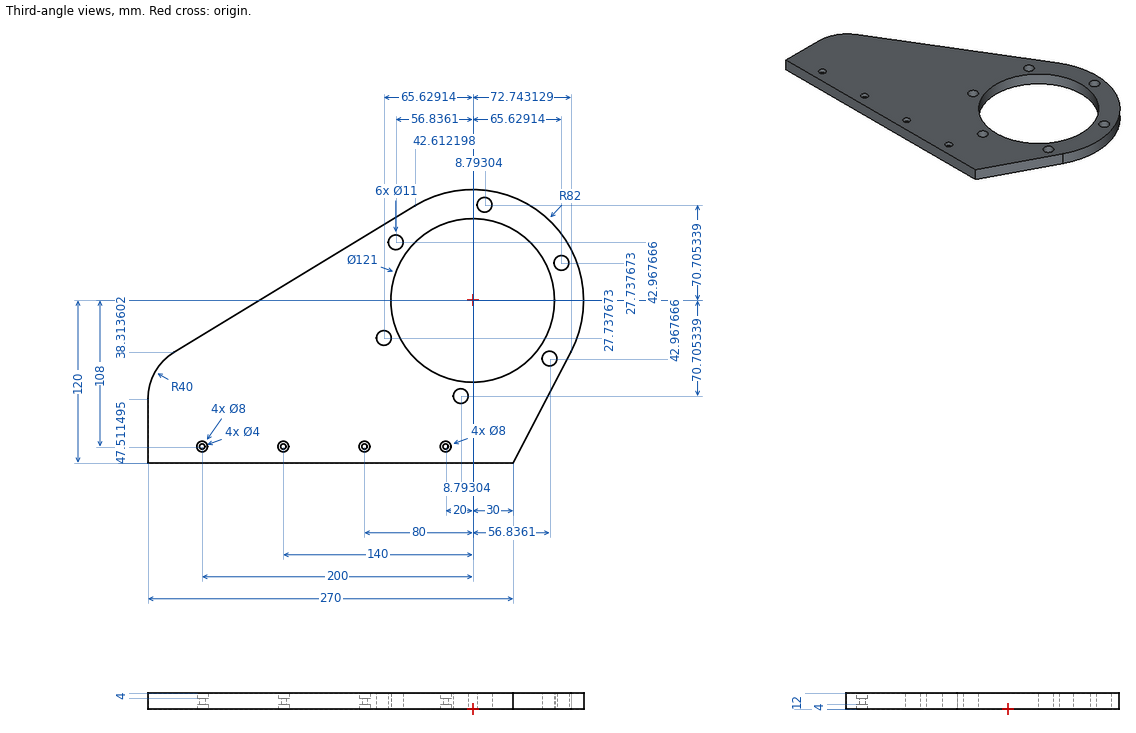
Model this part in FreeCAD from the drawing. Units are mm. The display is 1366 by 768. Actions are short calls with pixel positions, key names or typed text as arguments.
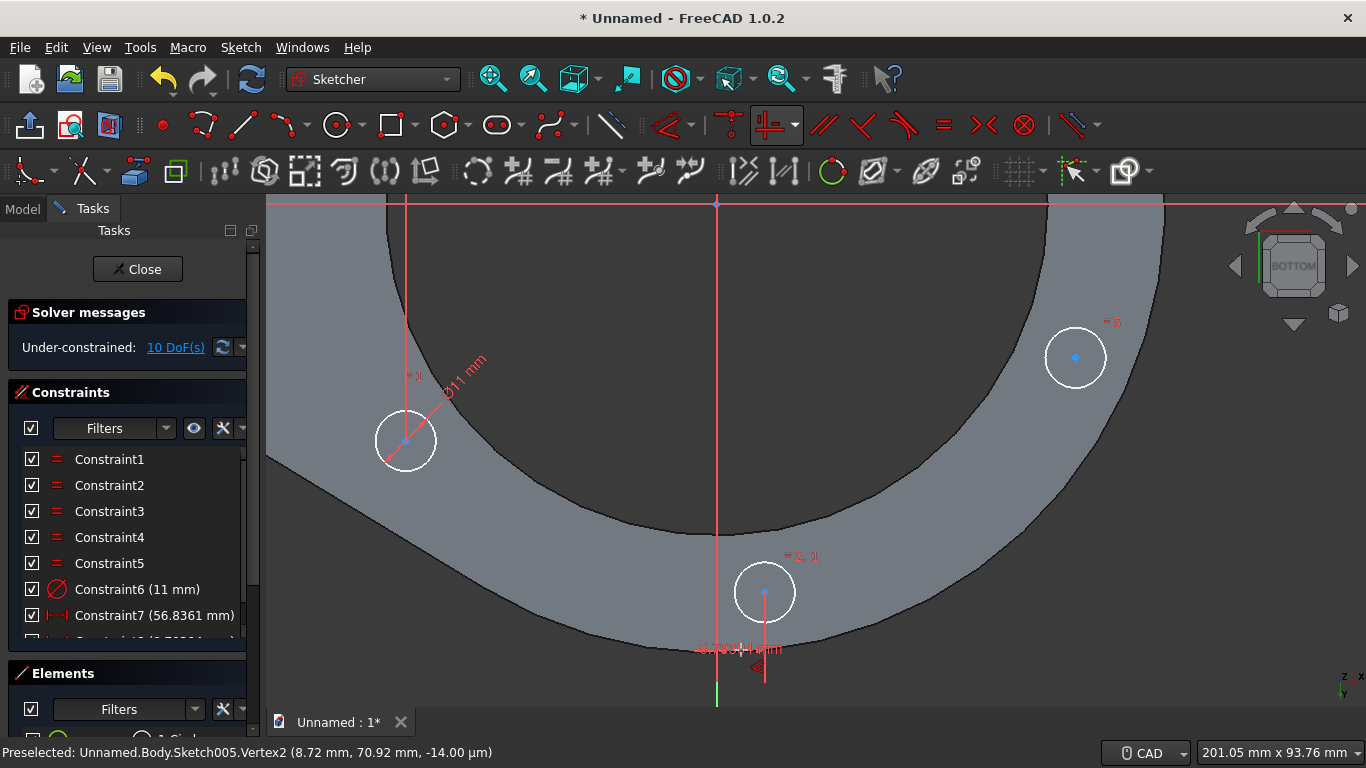
scroll(765, 594, down, 5)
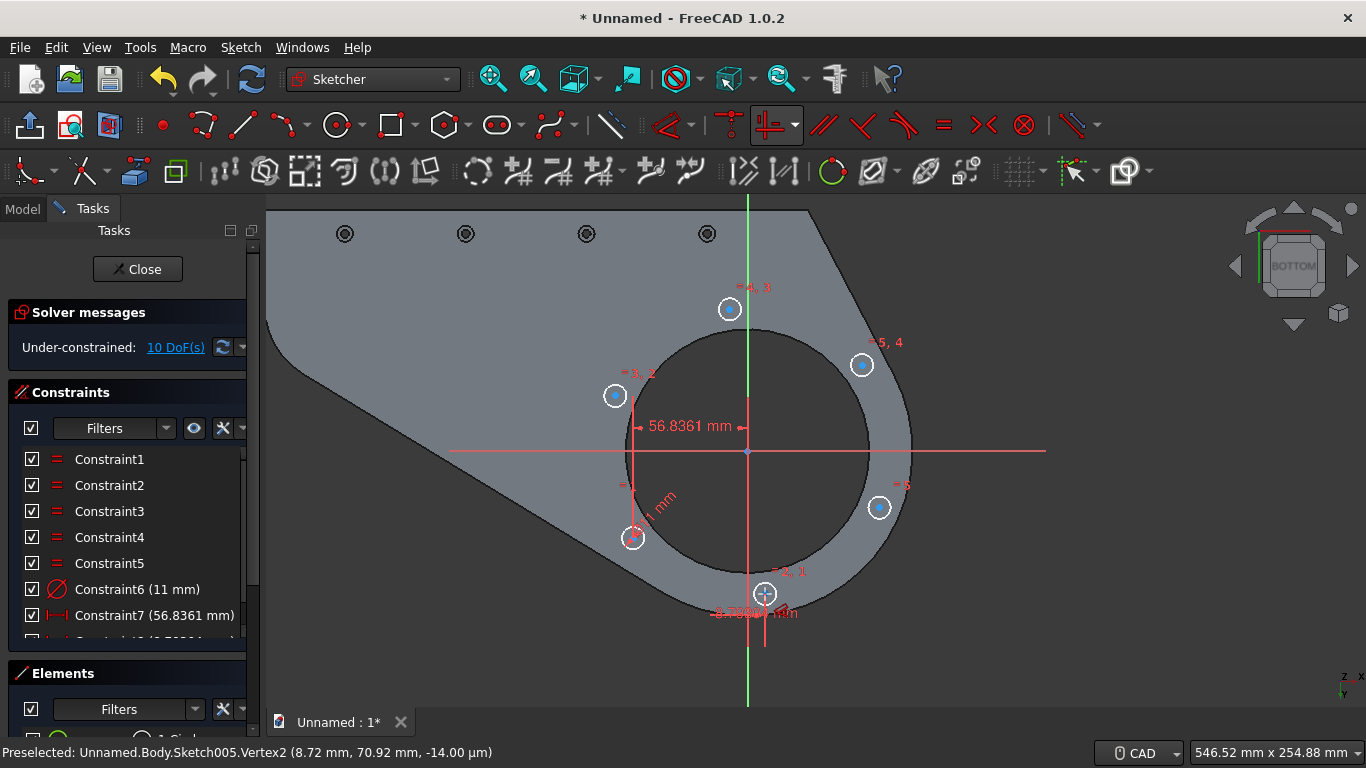
scroll(730, 309, up, 5)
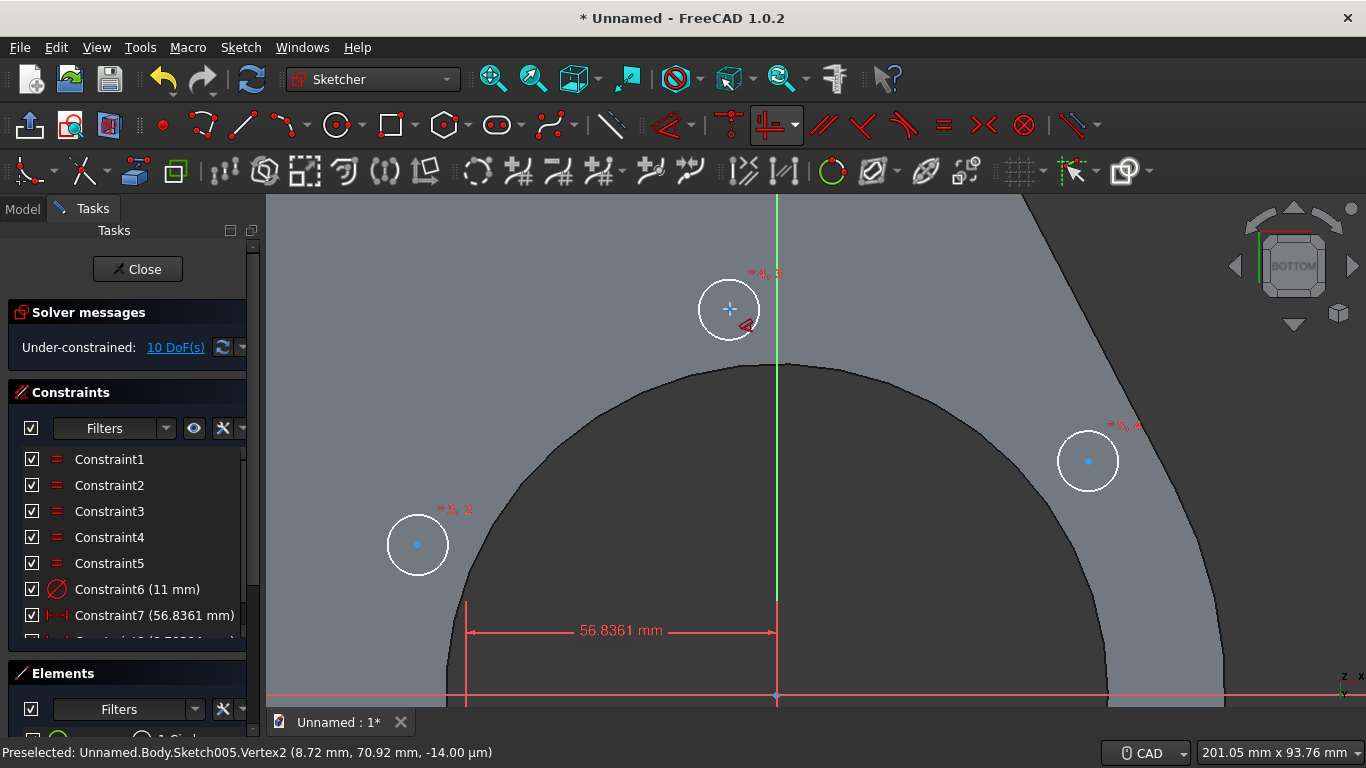
click(729, 310)
click(753, 252)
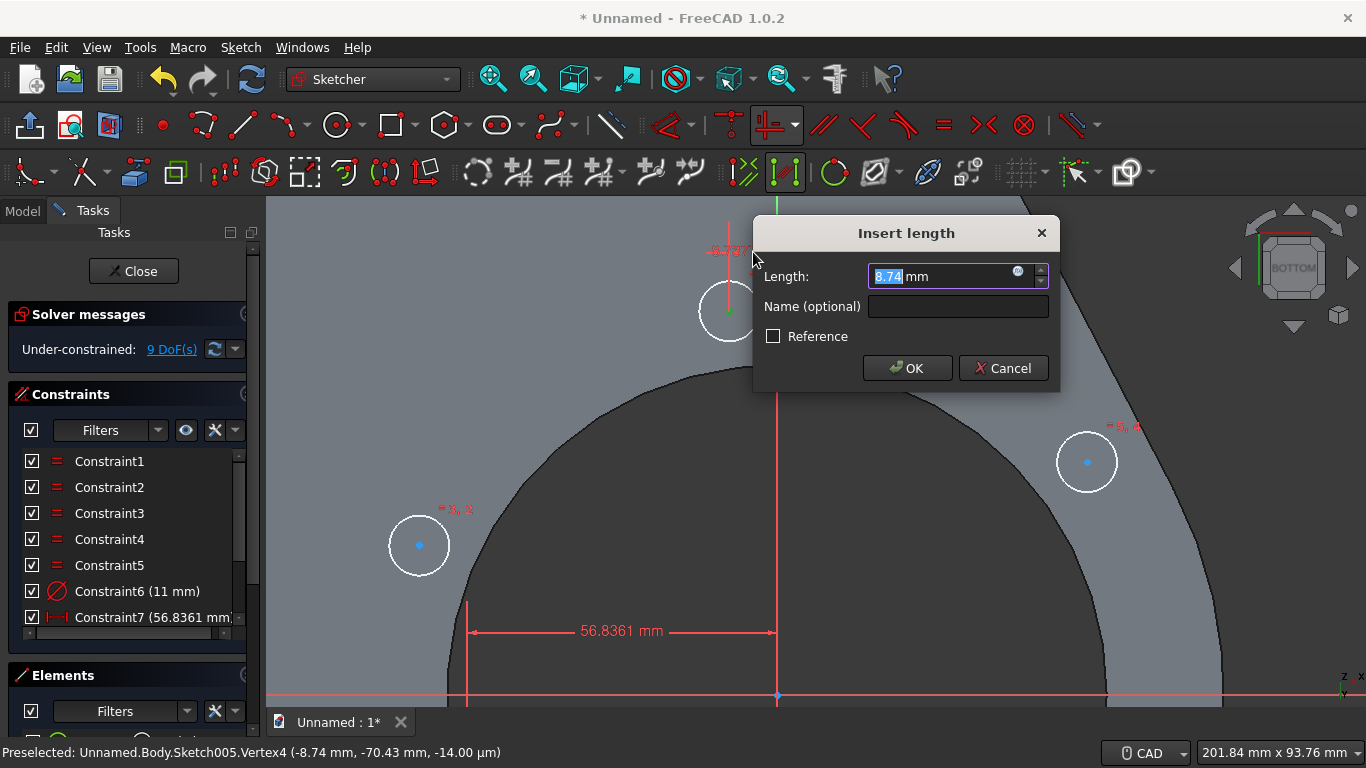
text(8.79304)
key(Return)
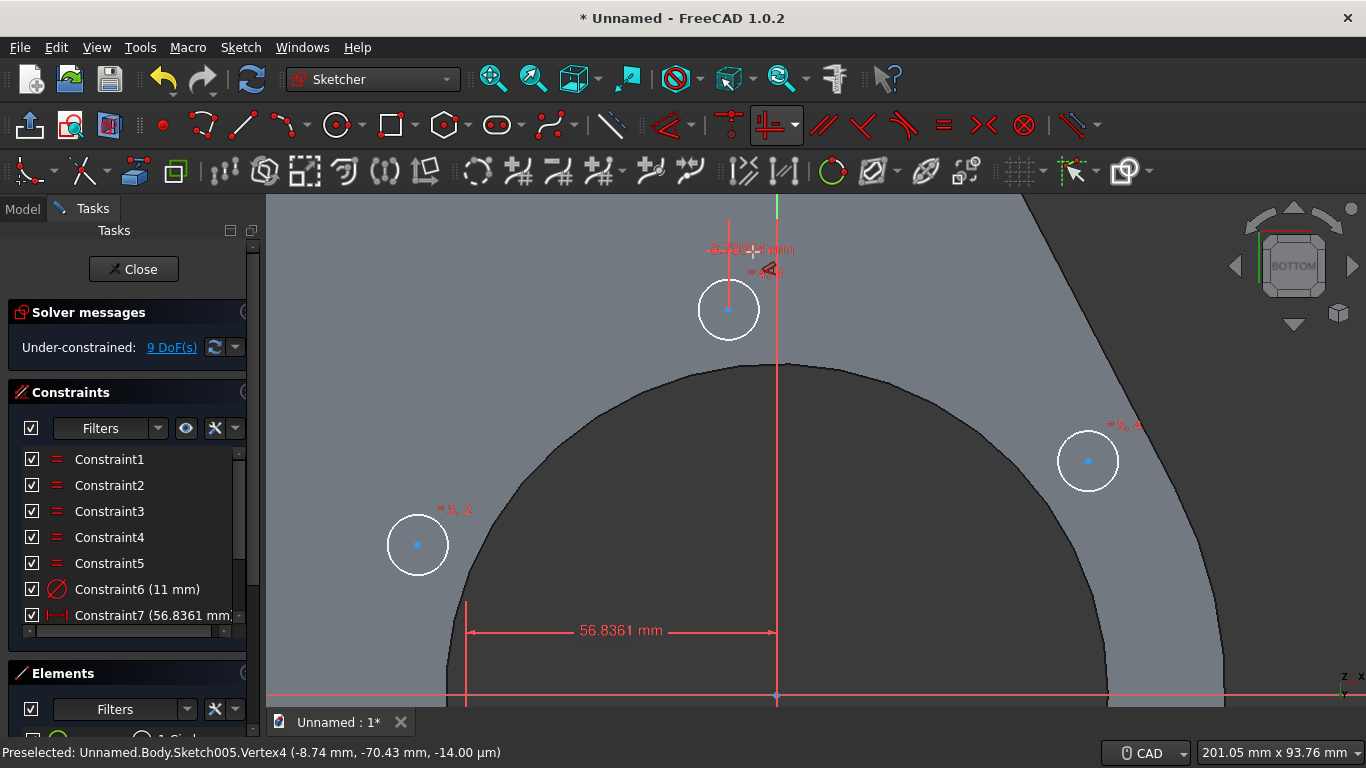
click(1088, 461)
click(933, 427)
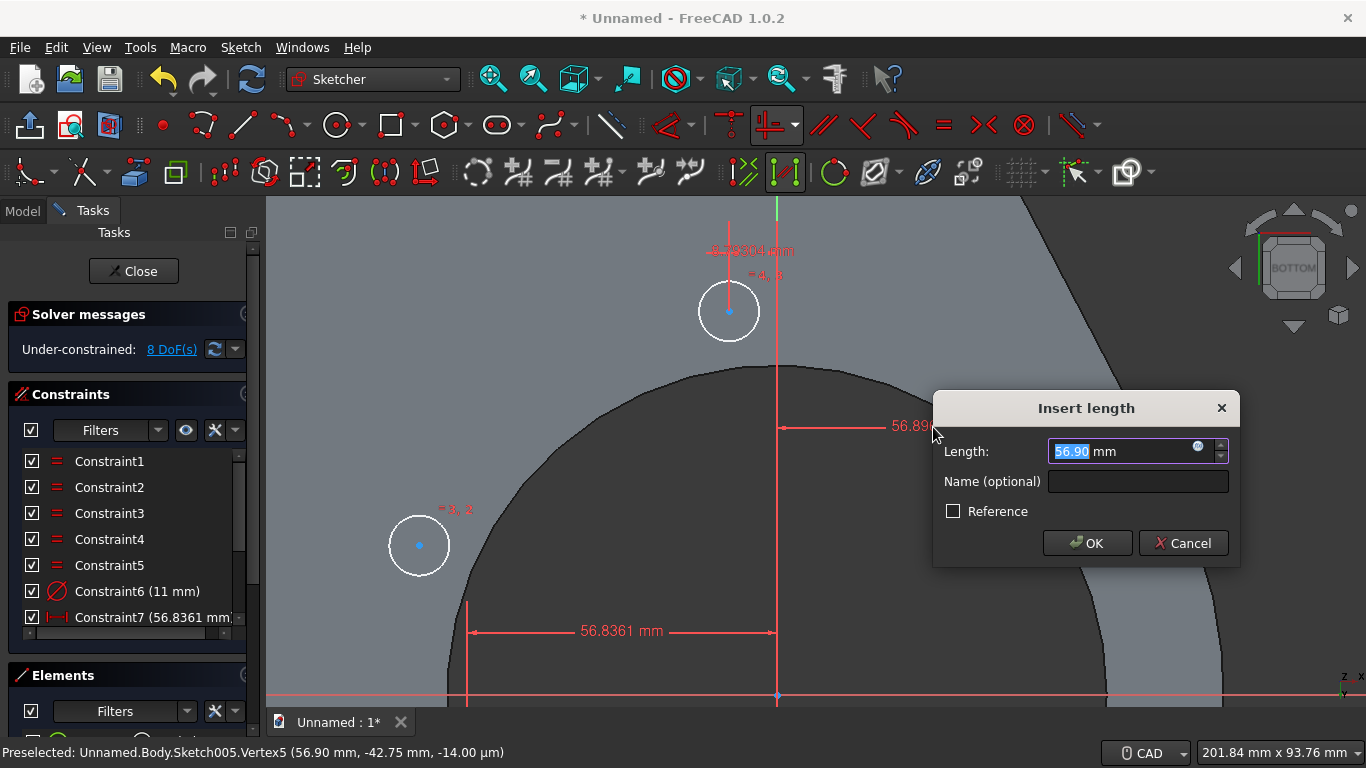
text(56.8361)
key(Return)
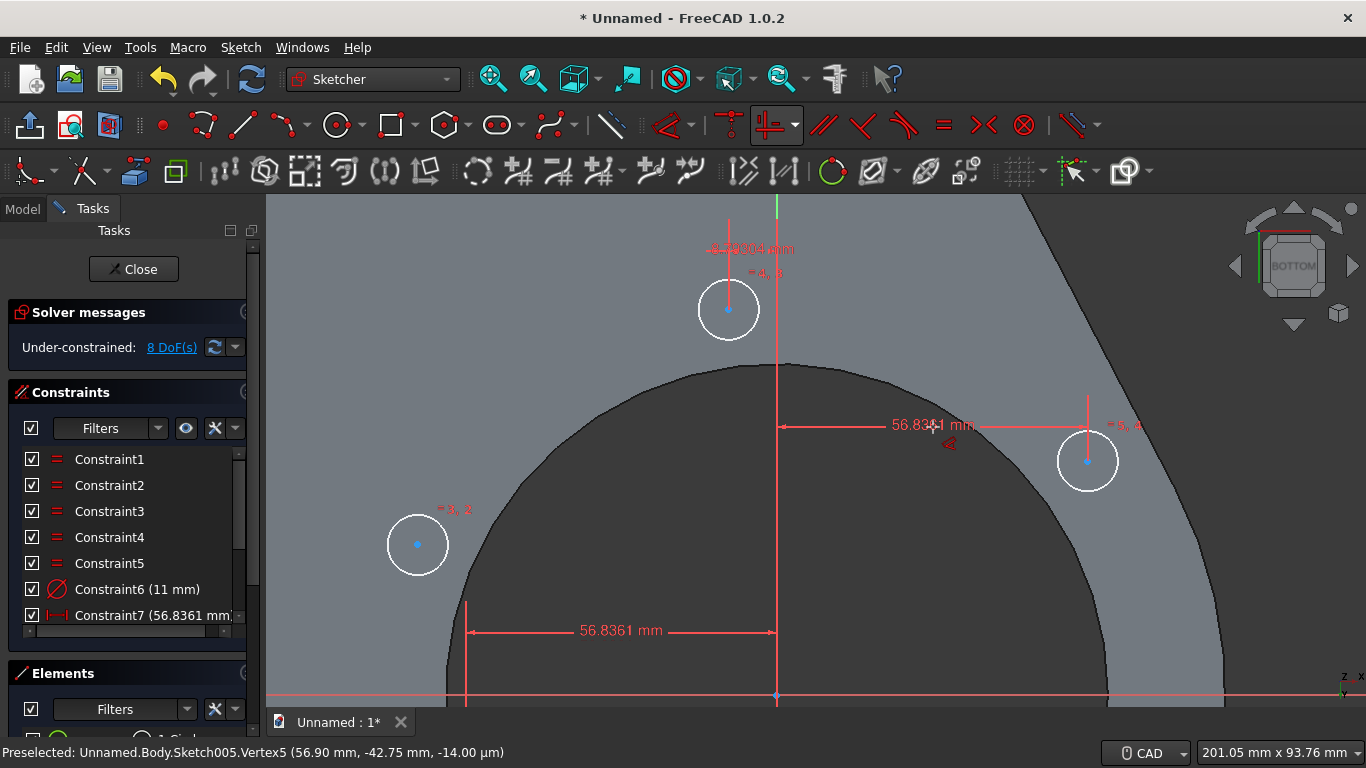
click(418, 545)
click(597, 511)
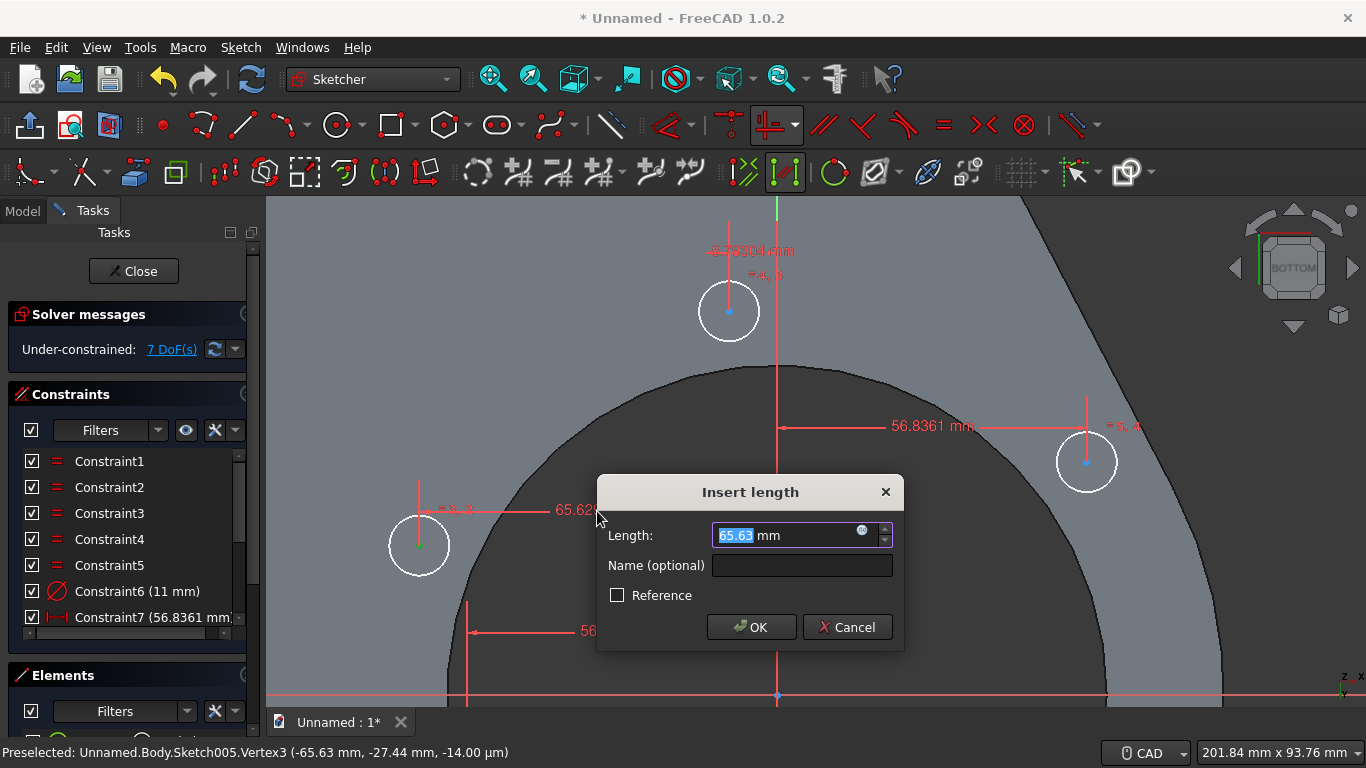
text(65.62914)
key(Return)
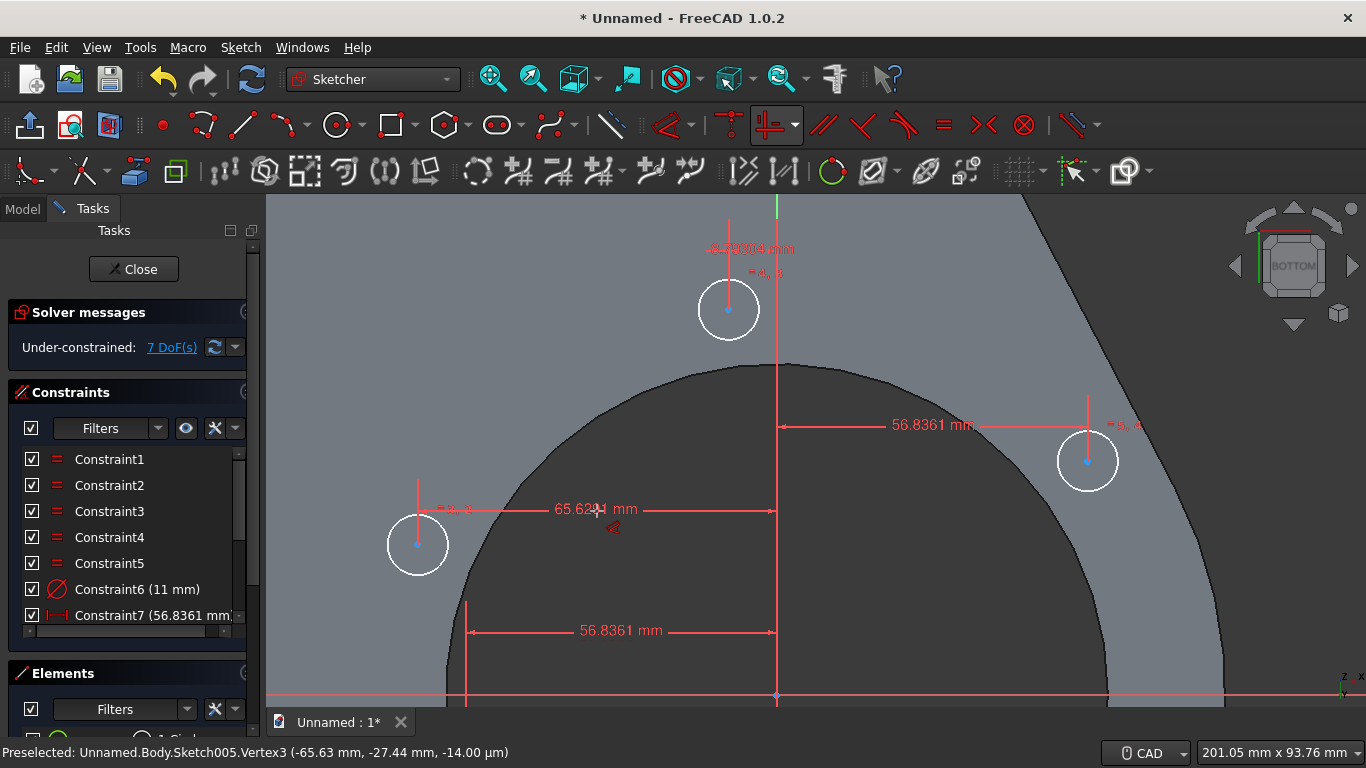
scroll(730, 308, down, 5)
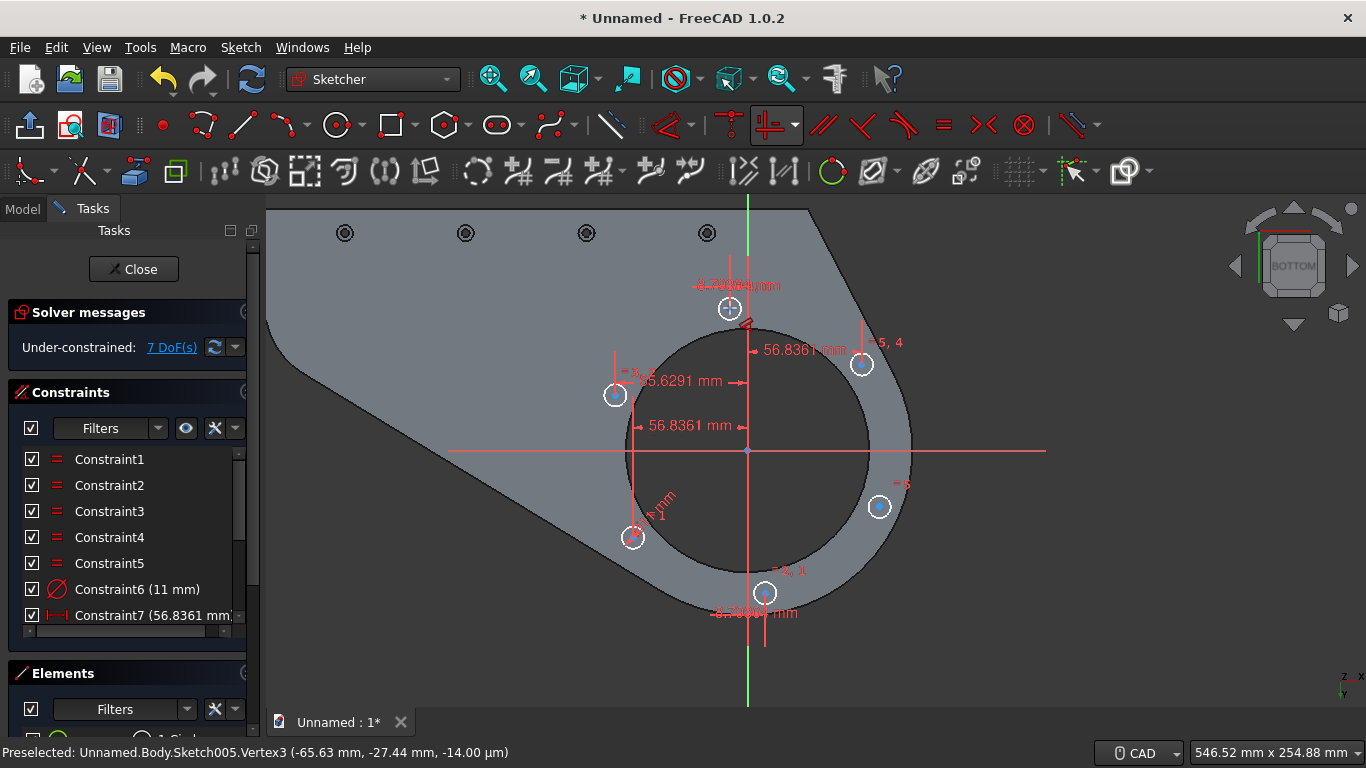
click(880, 507)
click(814, 541)